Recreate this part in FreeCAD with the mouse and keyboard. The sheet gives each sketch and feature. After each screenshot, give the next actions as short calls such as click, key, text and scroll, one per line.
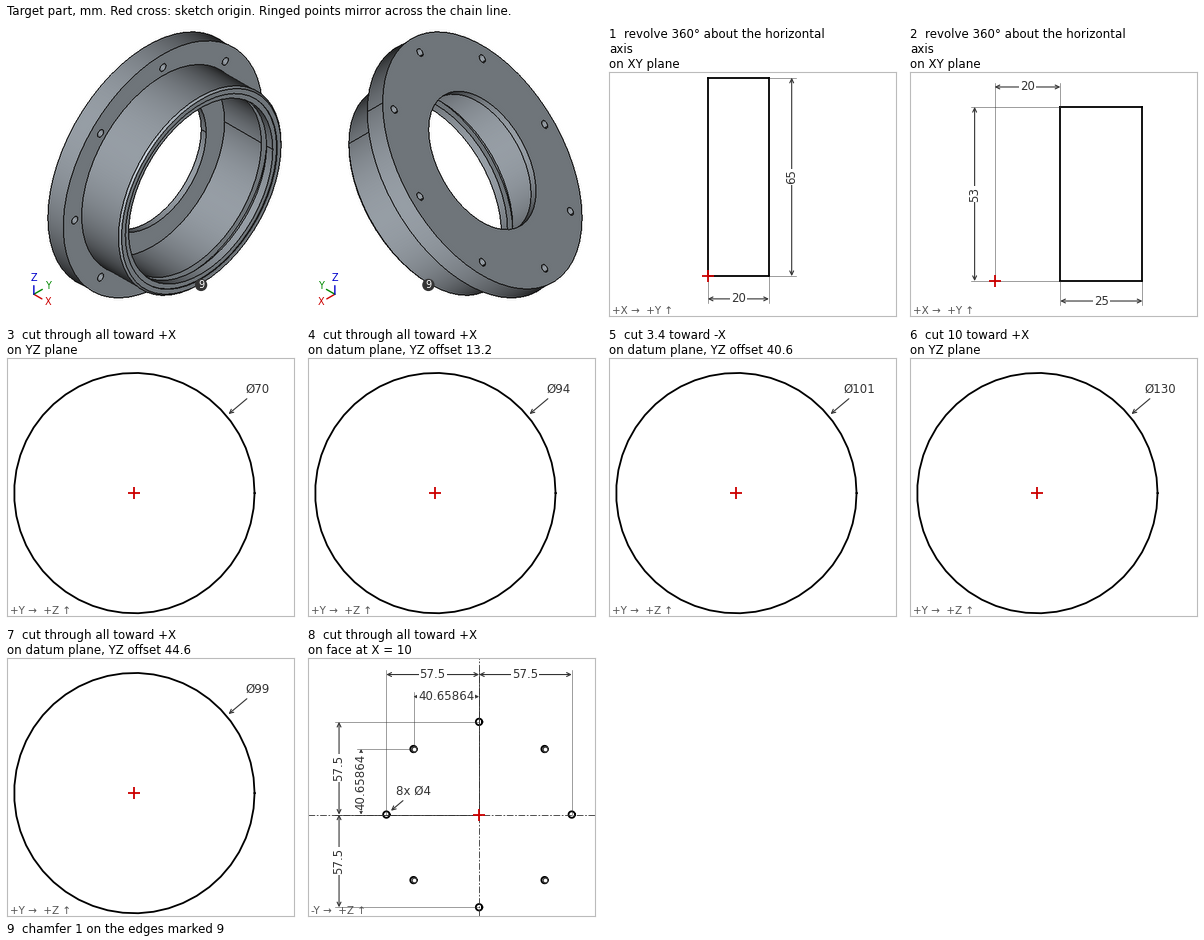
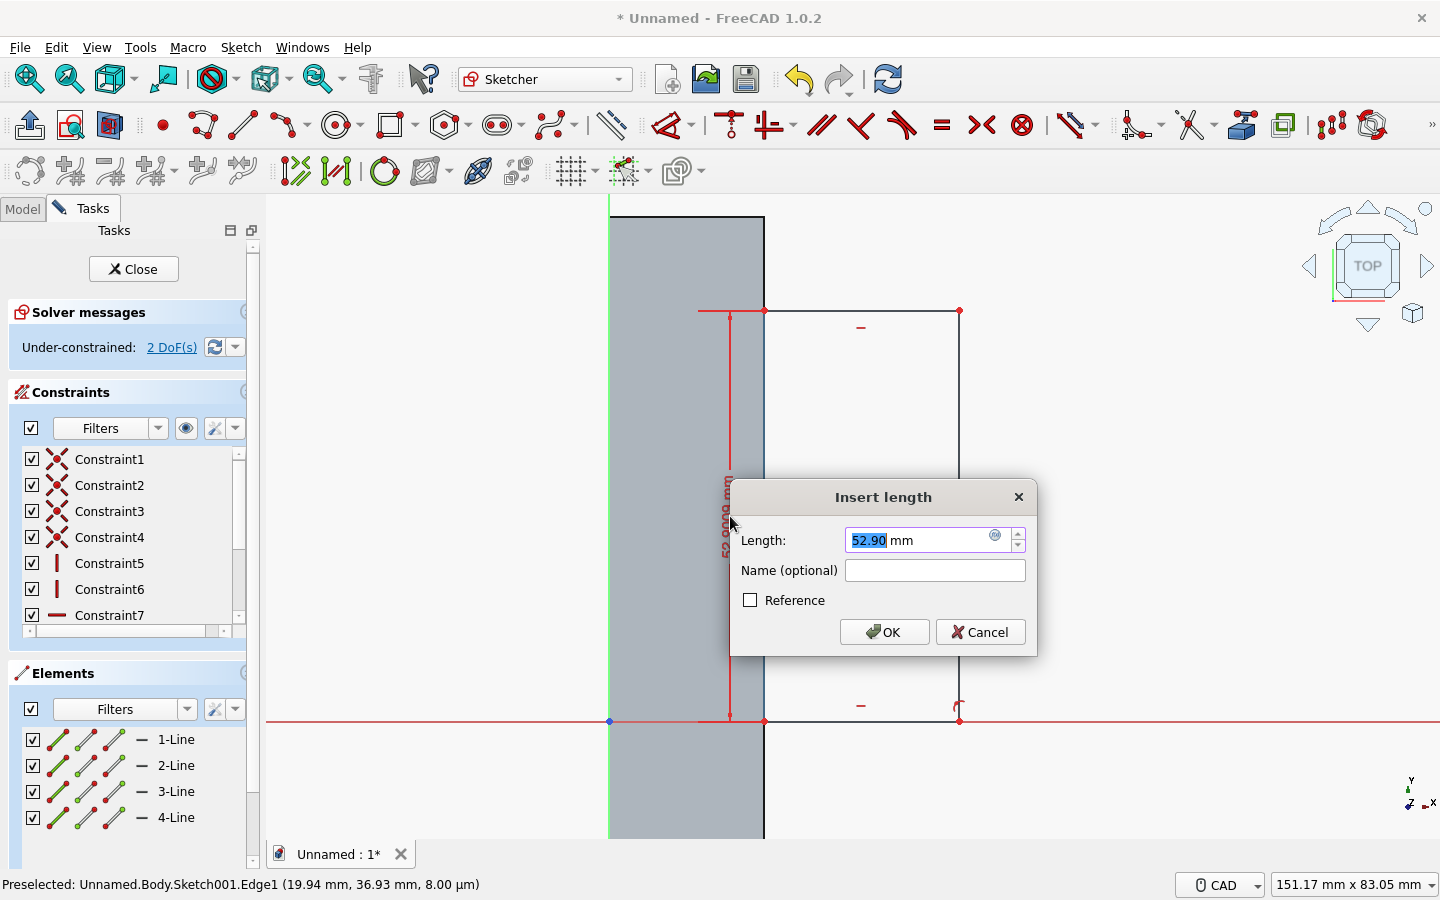
text(53)
key(Return)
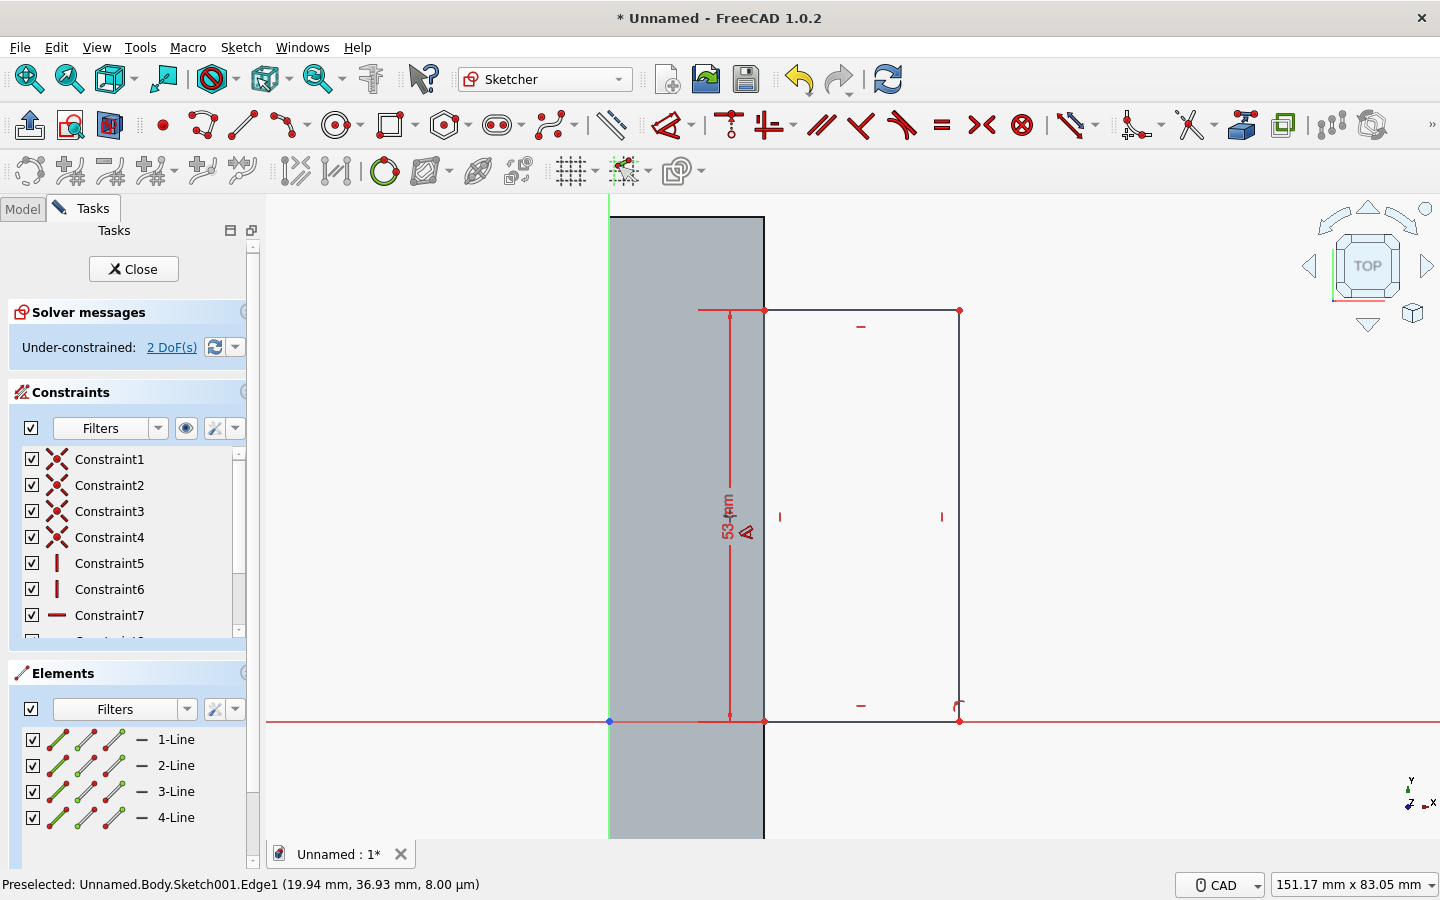
click(822, 722)
click(861, 756)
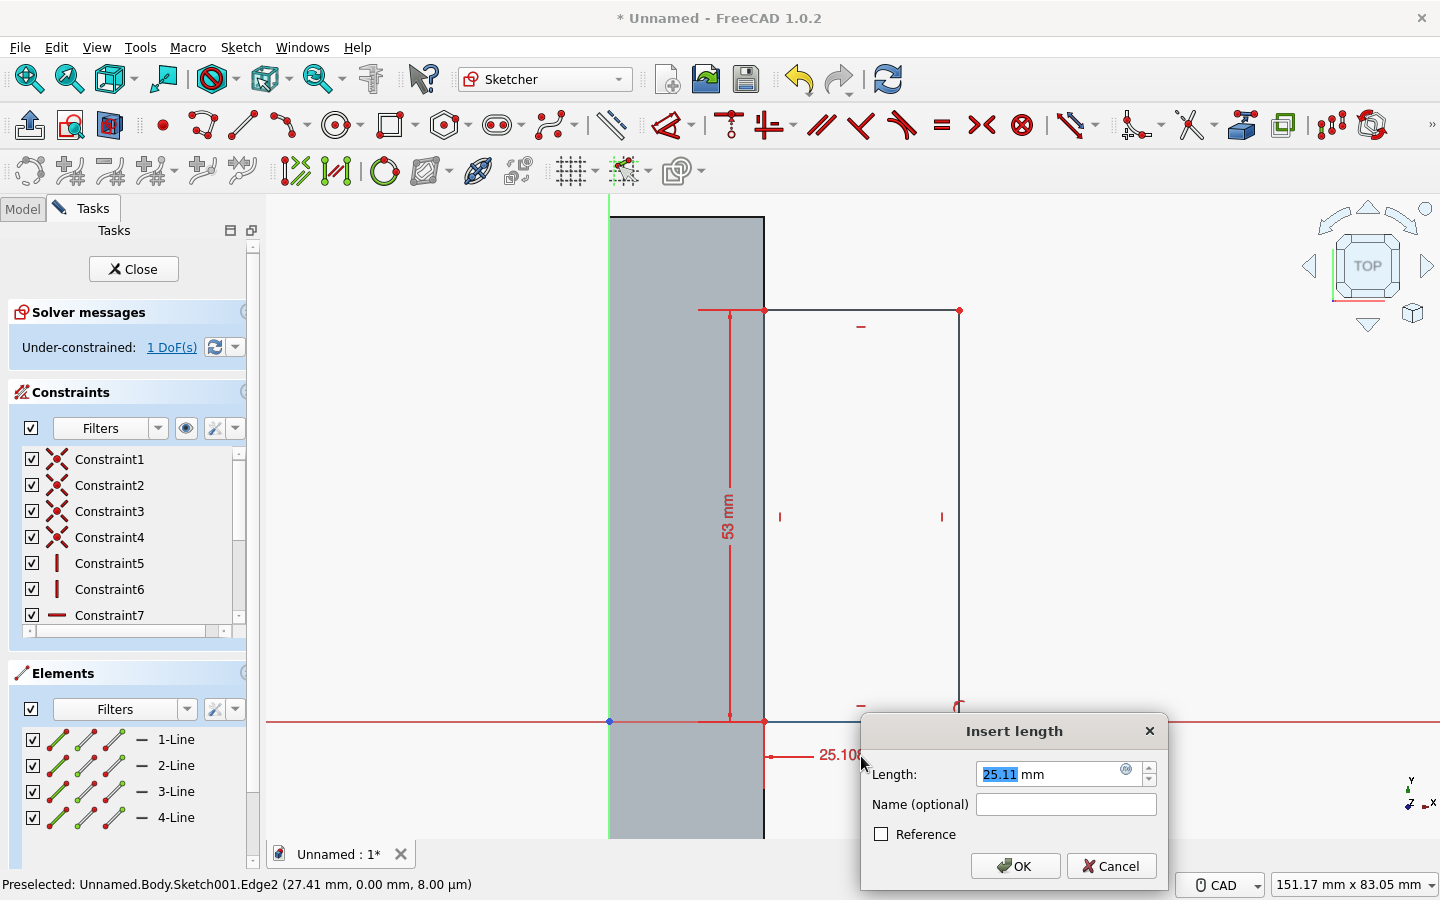
text(25)
key(Return)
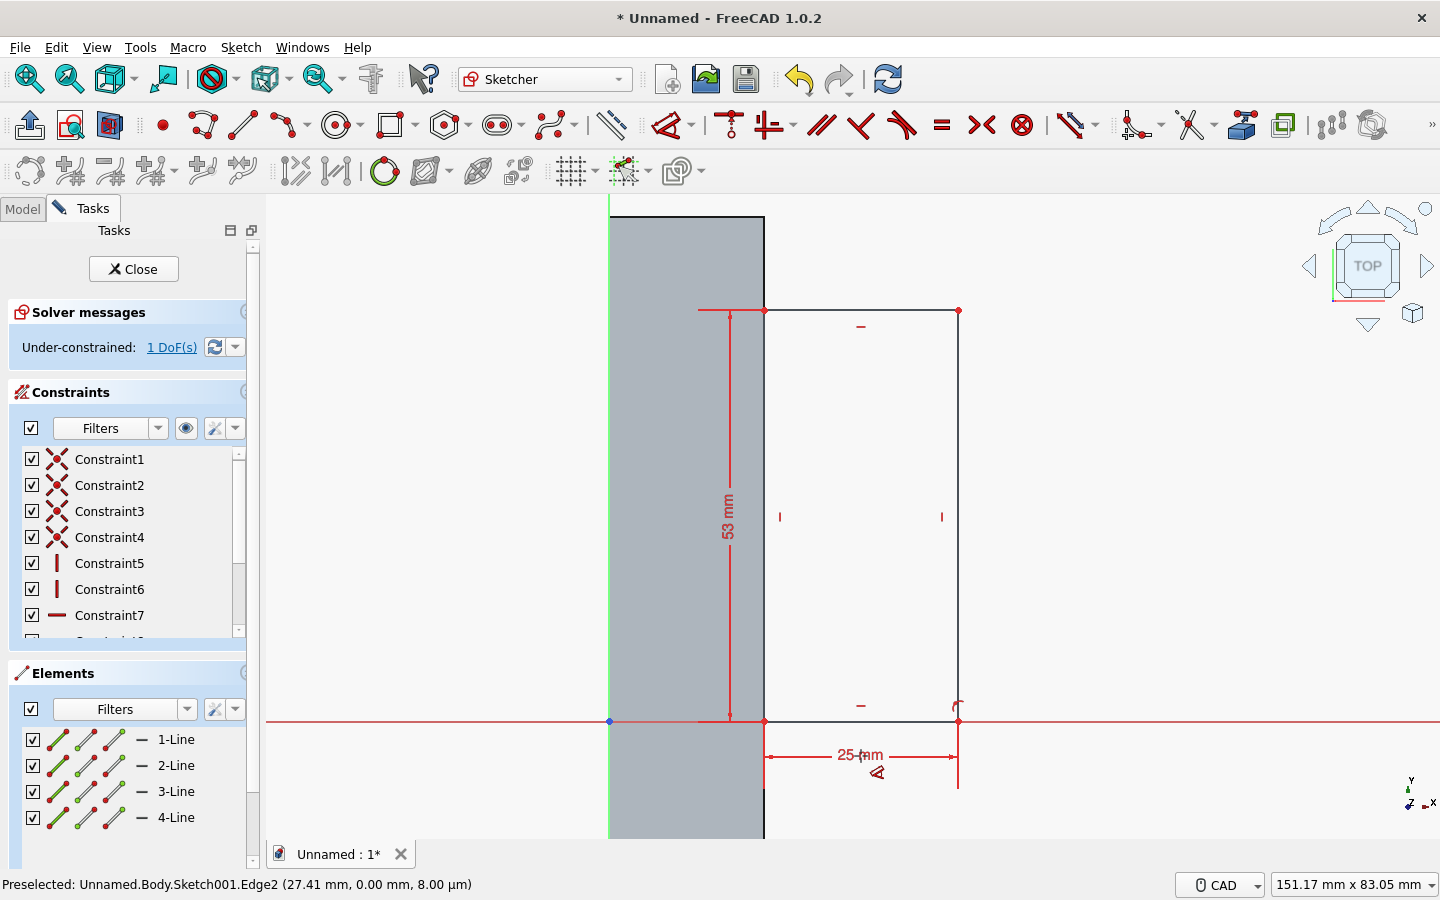
click(764, 310)
click(687, 756)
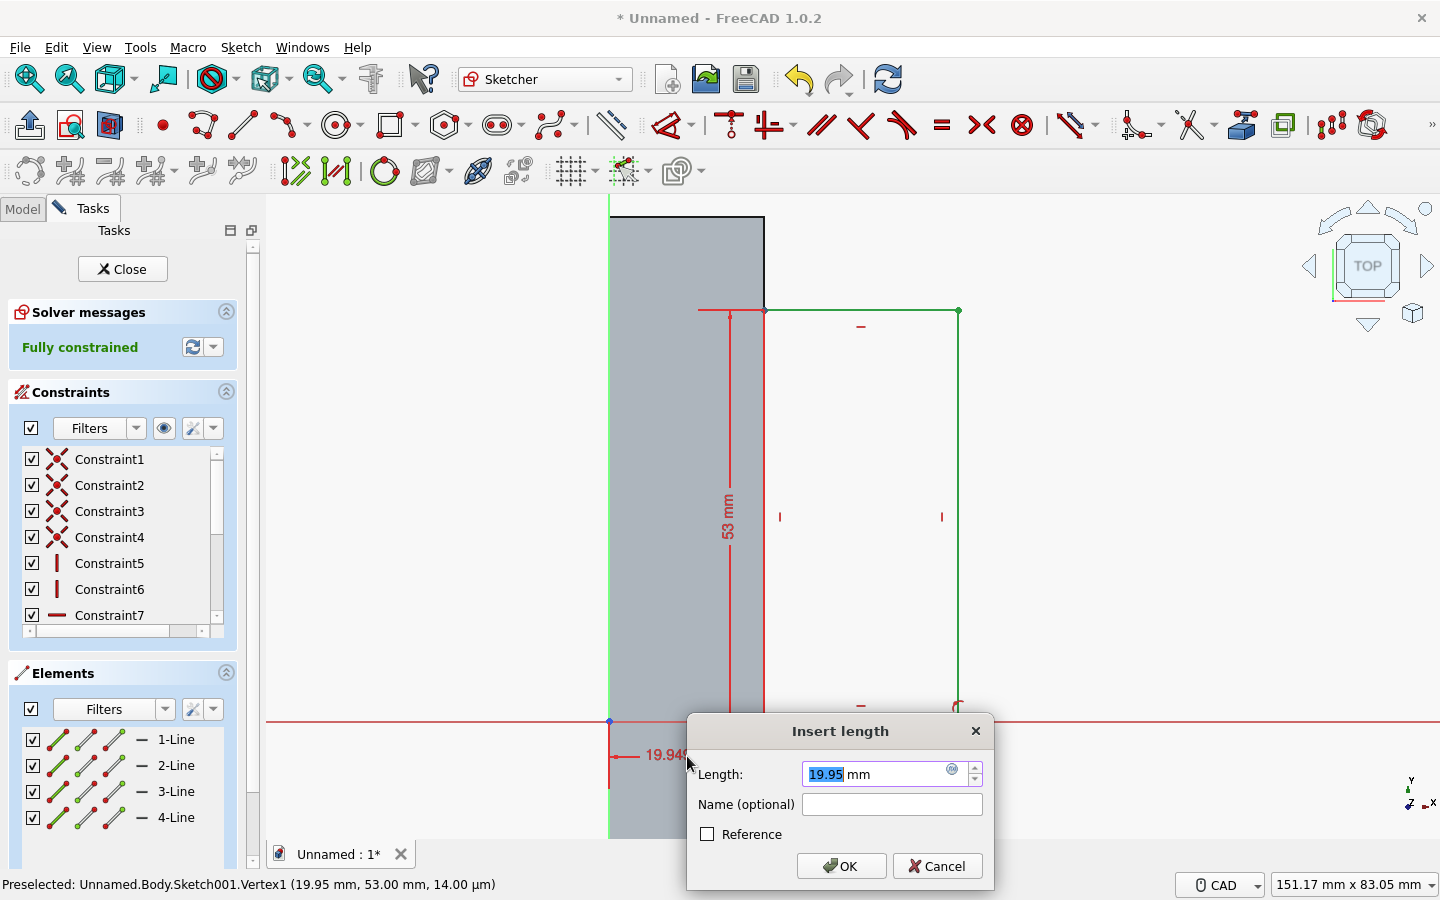
text(20)
key(Return)
key(Escape)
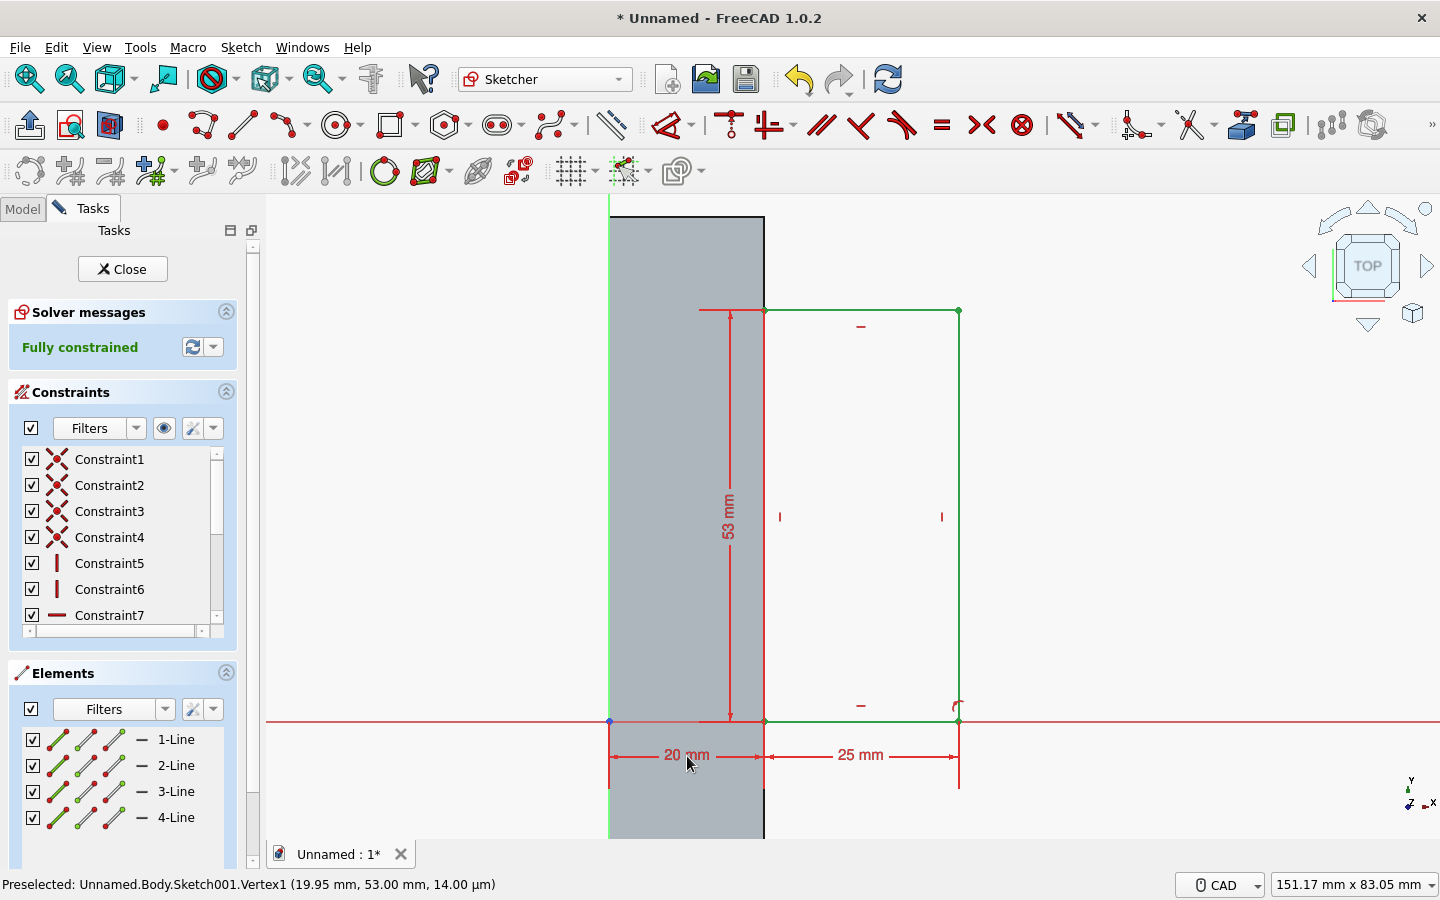
click(123, 269)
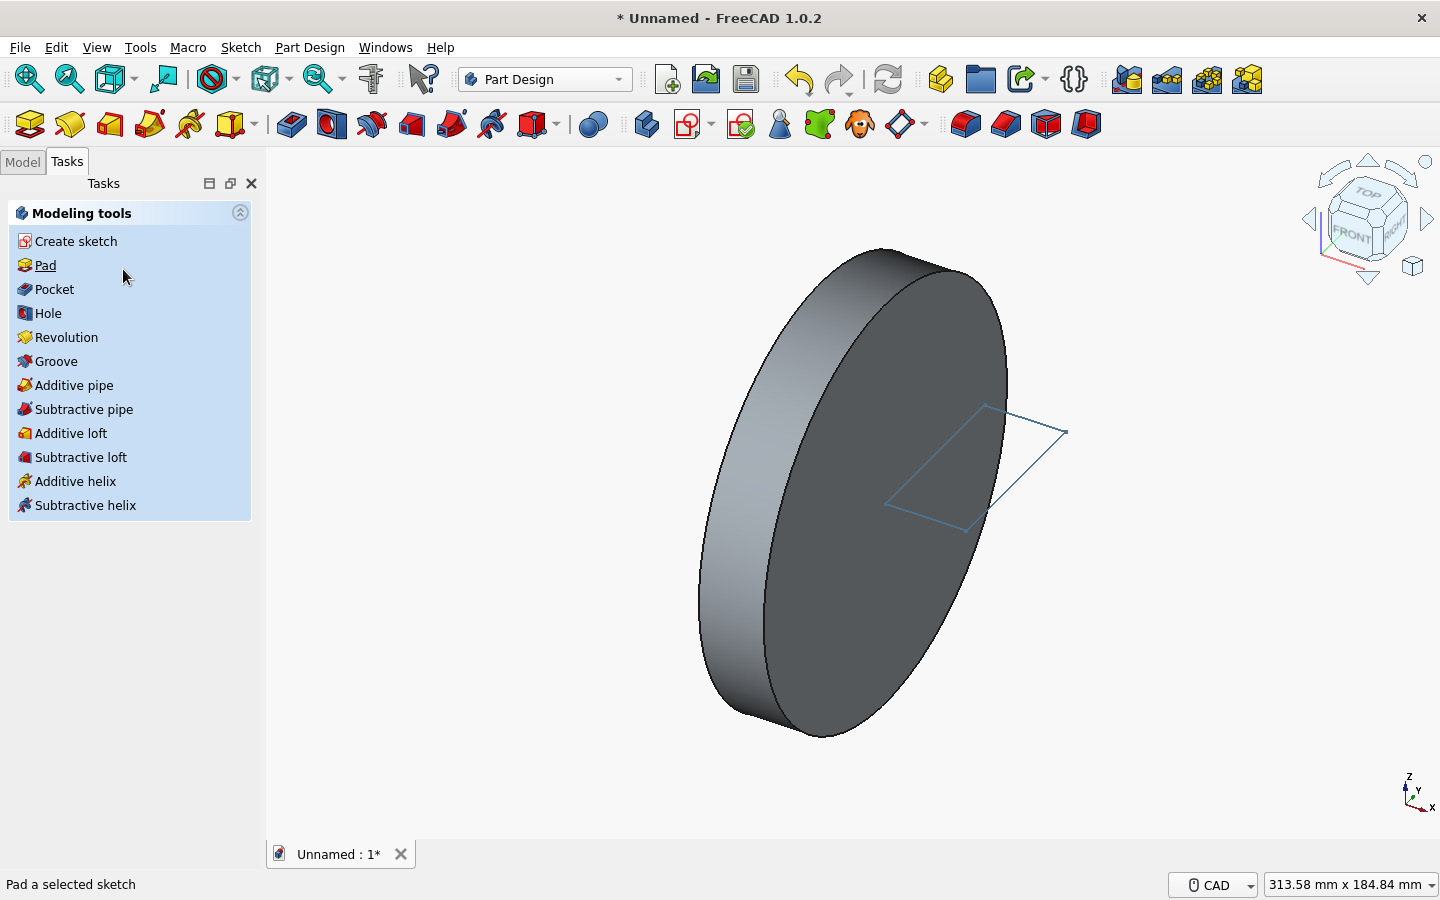
click(70, 124)